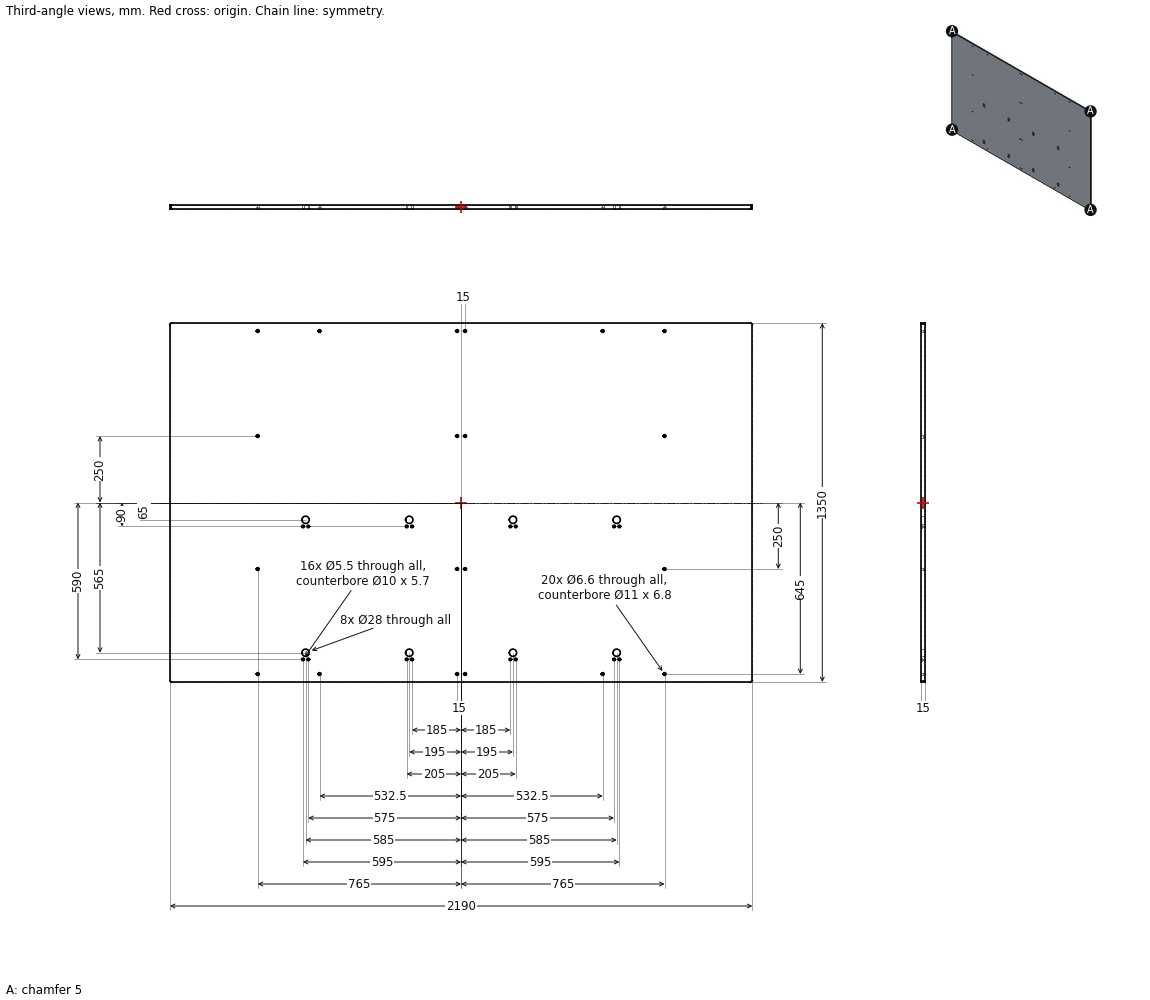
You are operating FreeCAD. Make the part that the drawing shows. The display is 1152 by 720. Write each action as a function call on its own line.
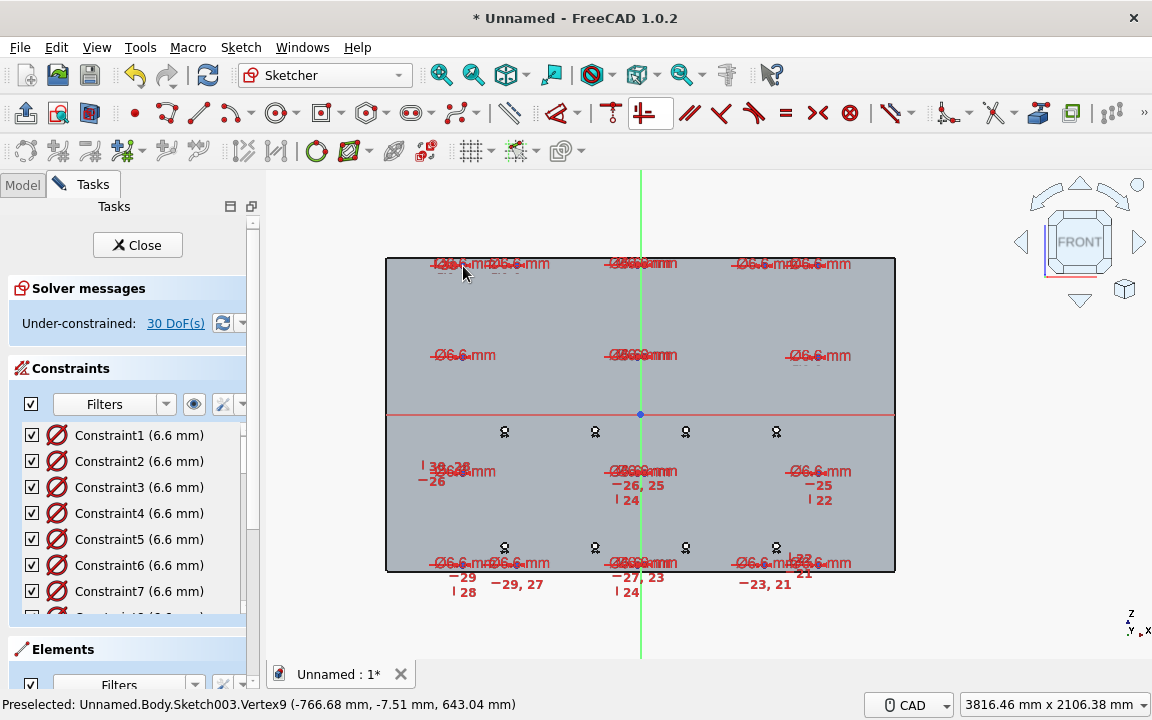
click(517, 565)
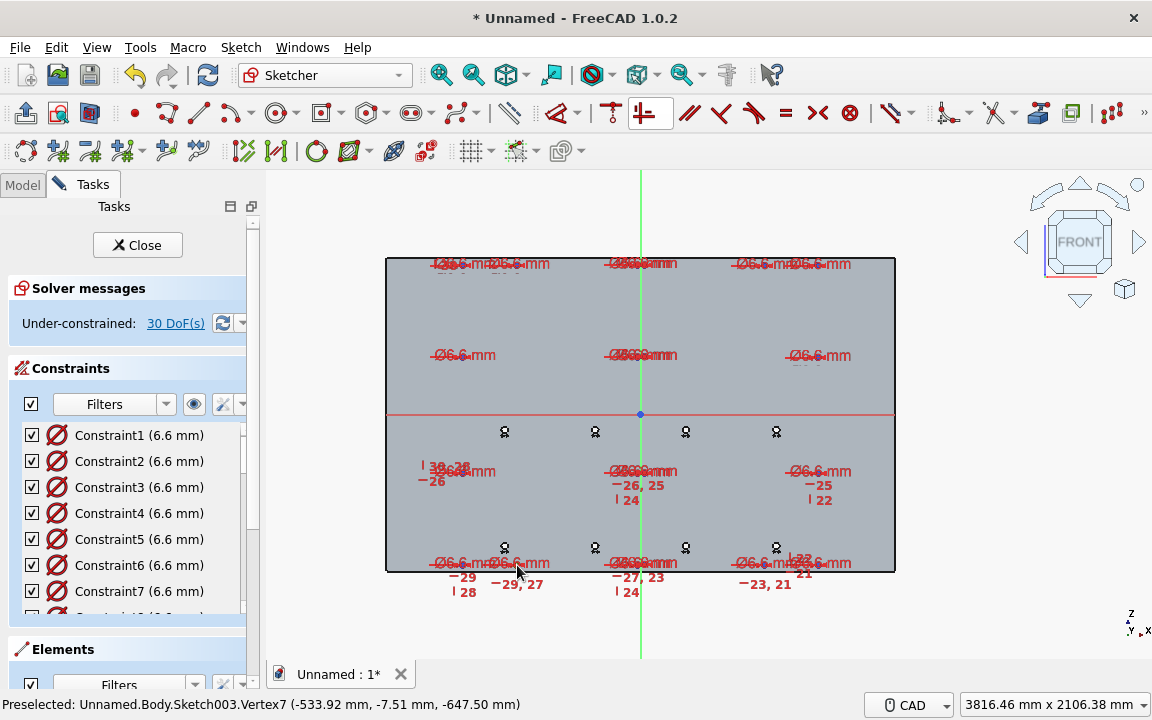
click(517, 266)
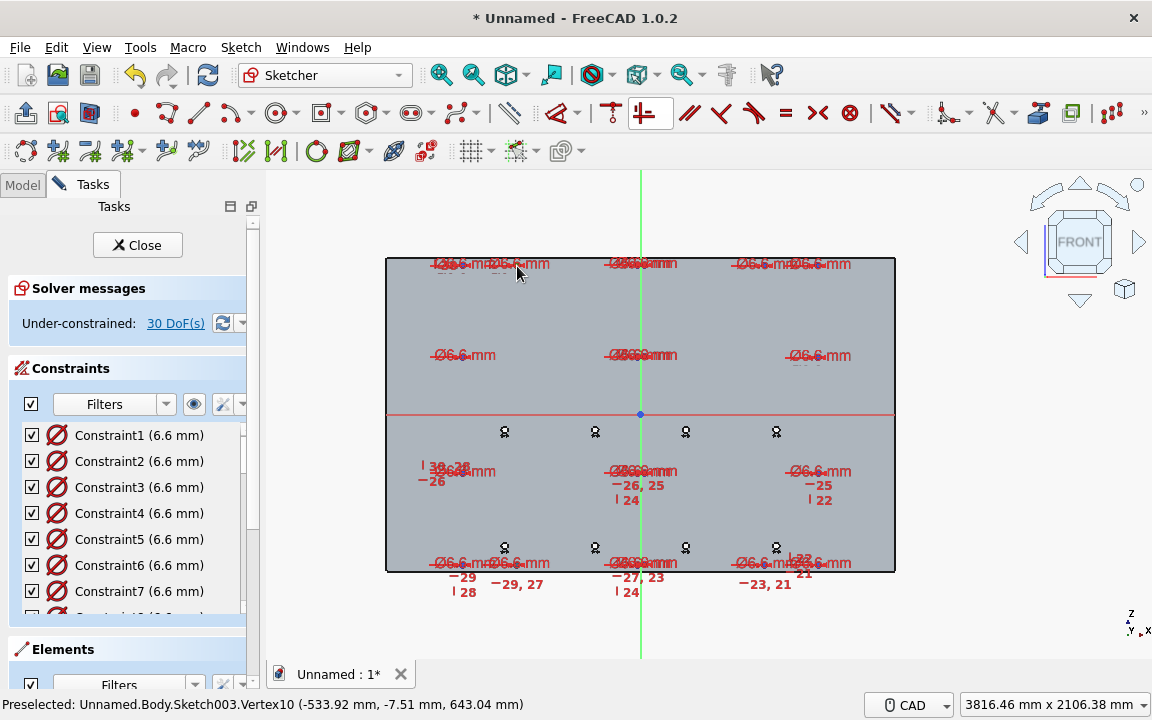
key(v)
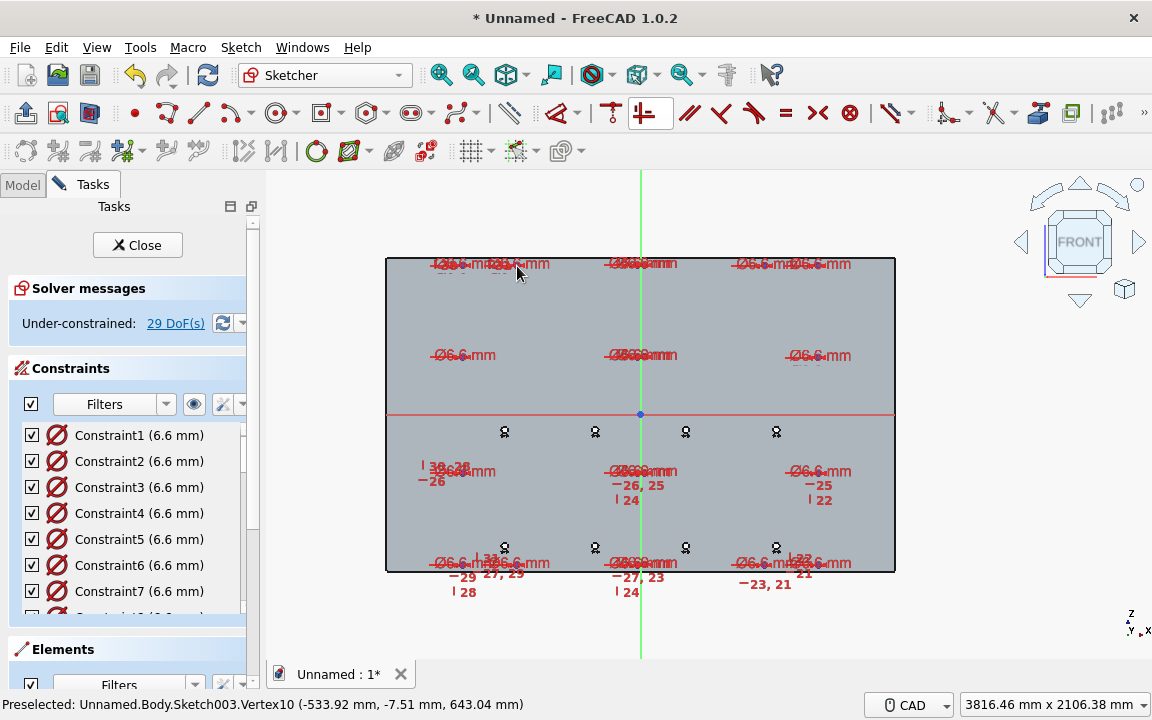
click(463, 266)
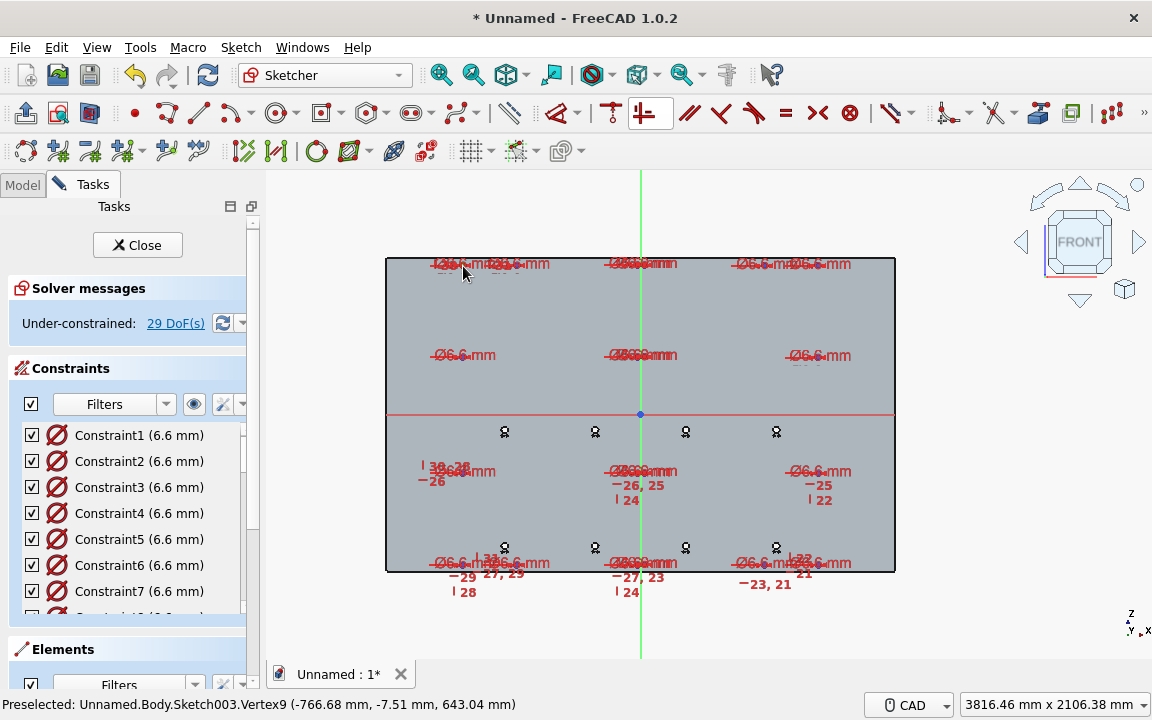
click(517, 266)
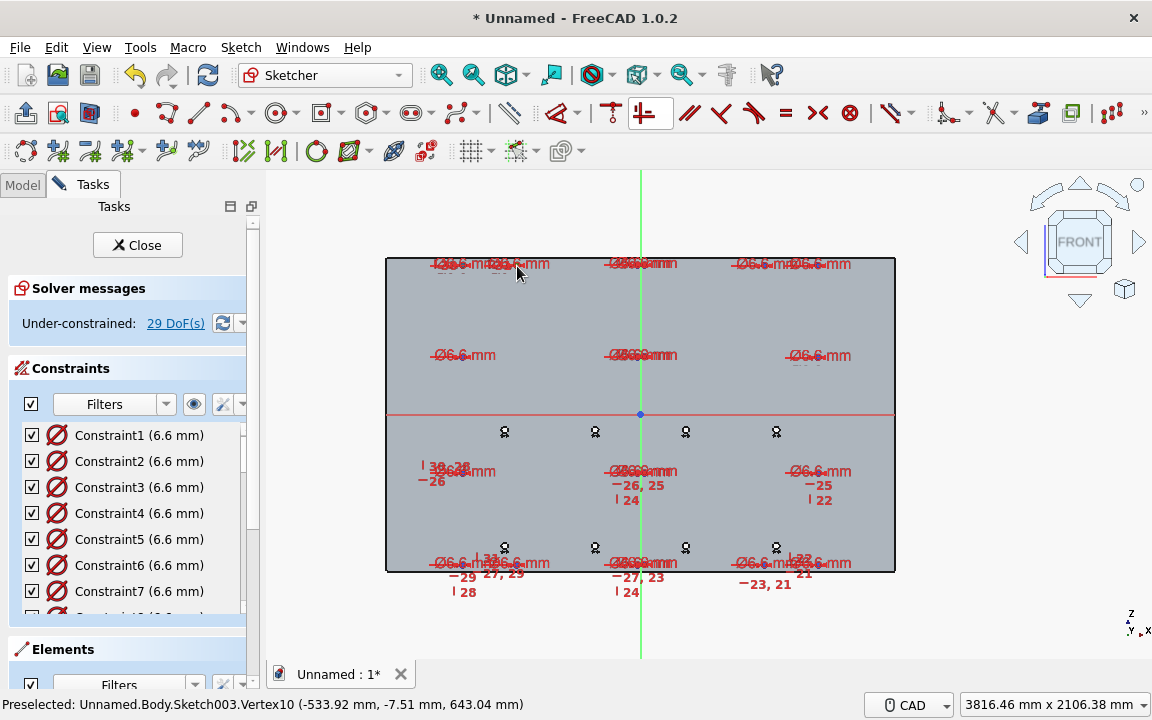
key(h)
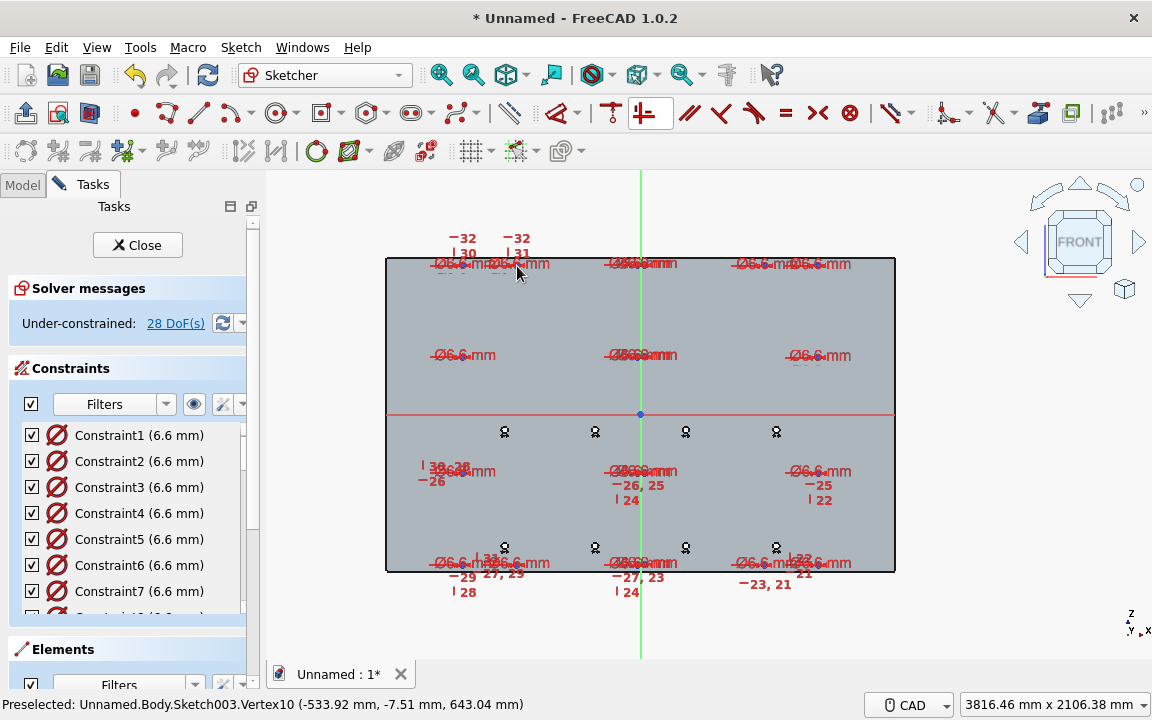
click(463, 266)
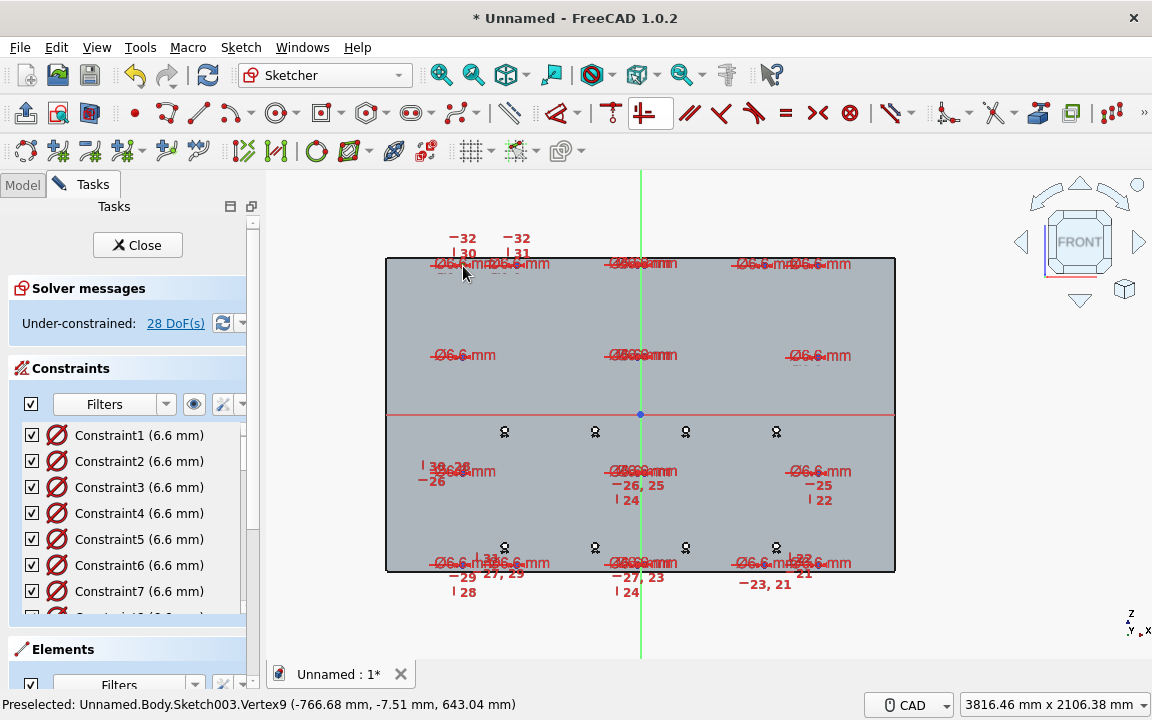
click(463, 357)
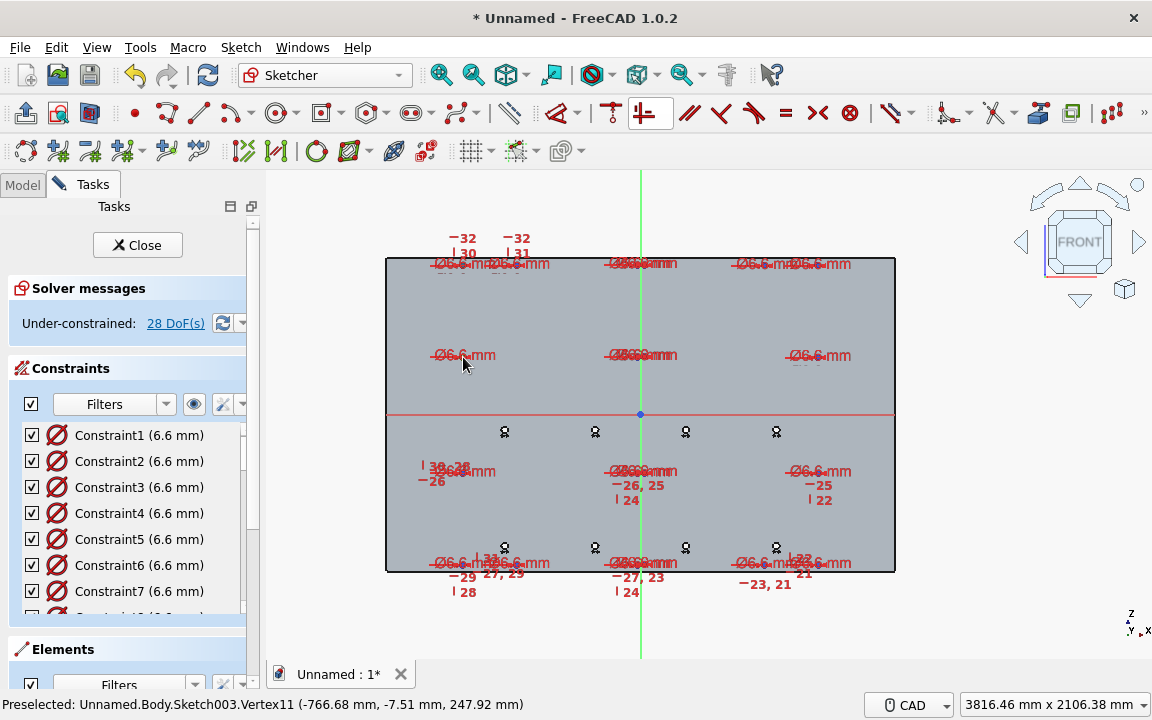
key(v)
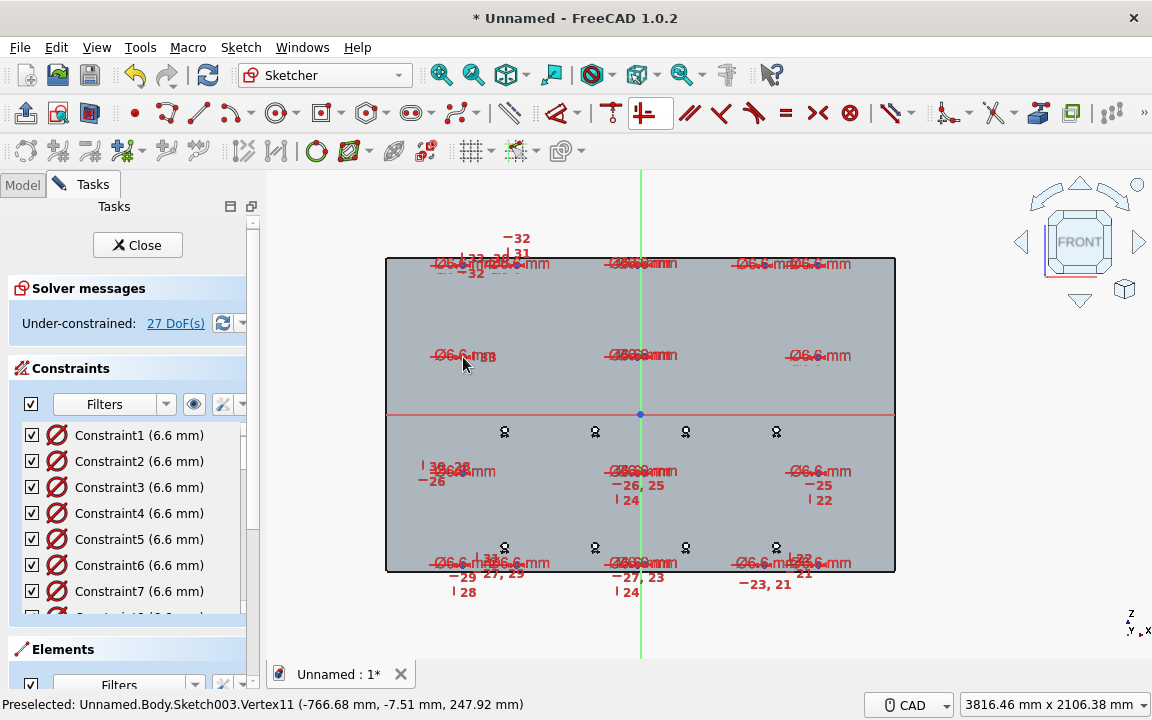
scroll(637, 473, up, 3)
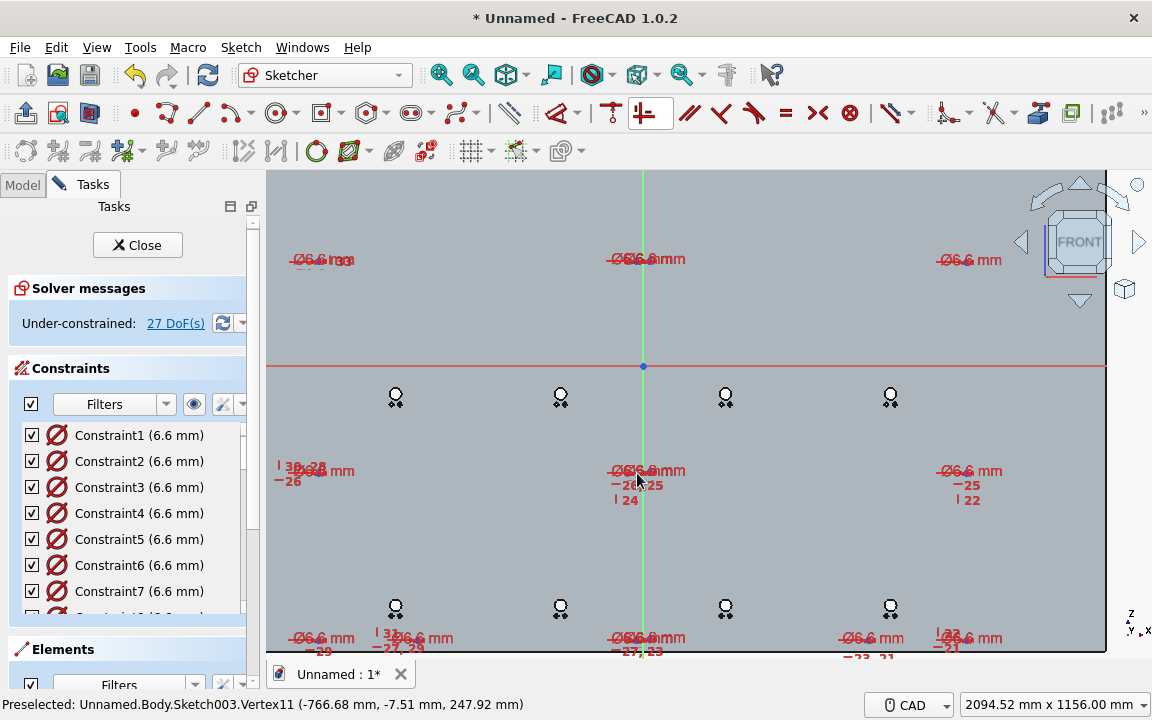
click(637, 473)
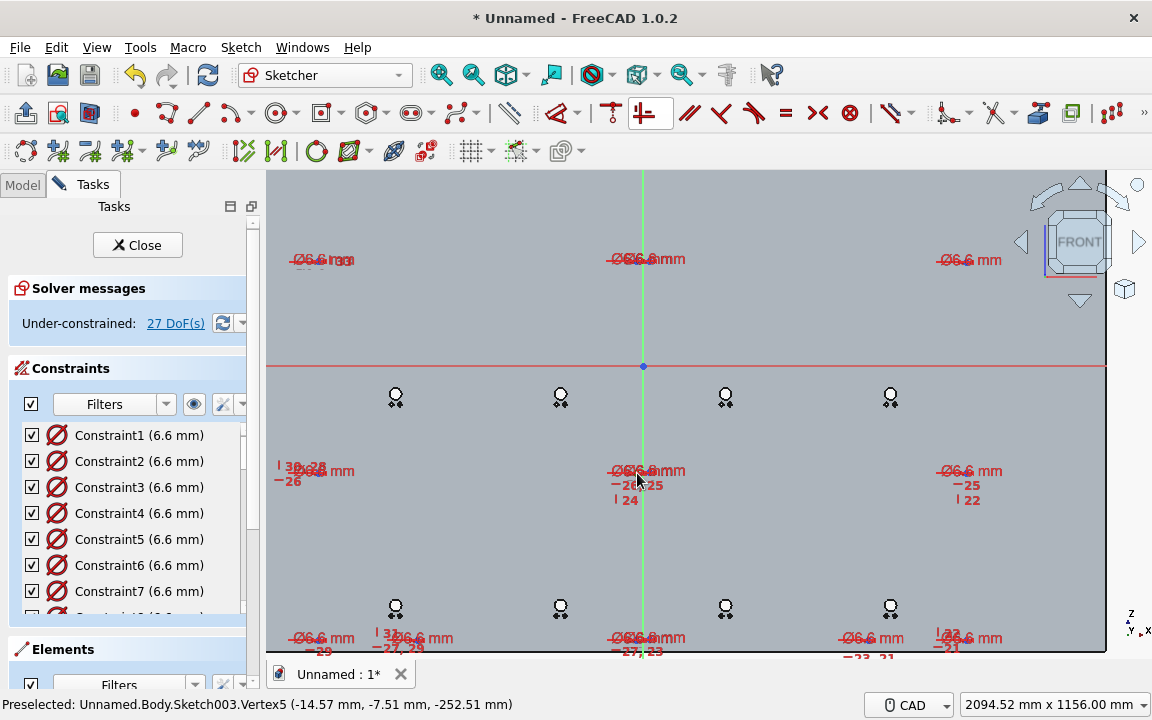
click(637, 261)